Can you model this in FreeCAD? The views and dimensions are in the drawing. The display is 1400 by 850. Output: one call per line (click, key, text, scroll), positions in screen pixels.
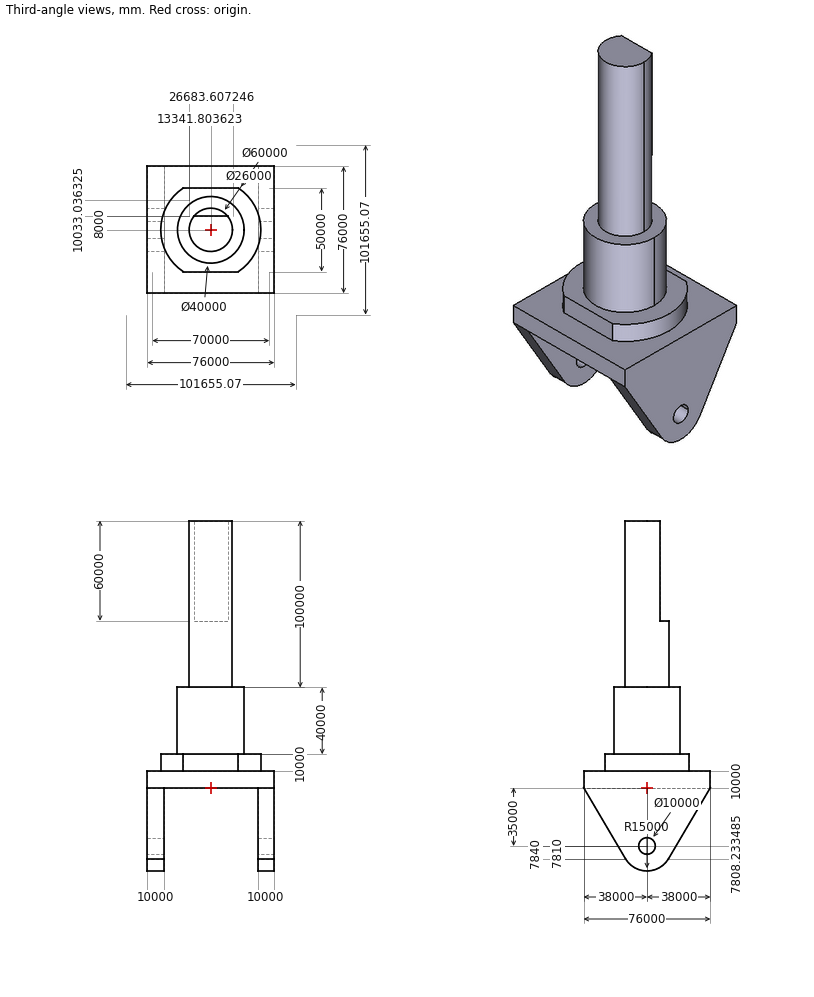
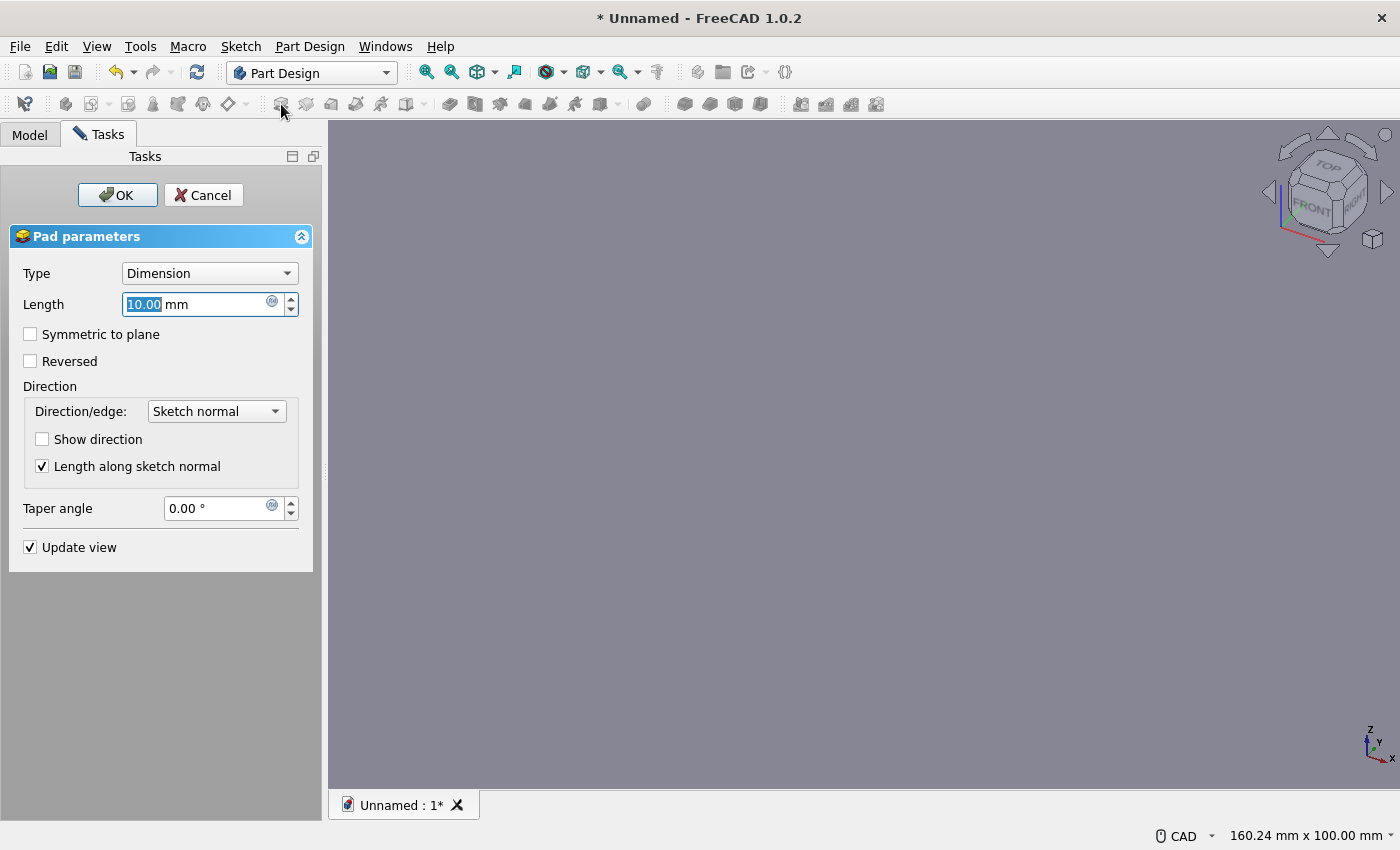
text(10000)
key(Tab)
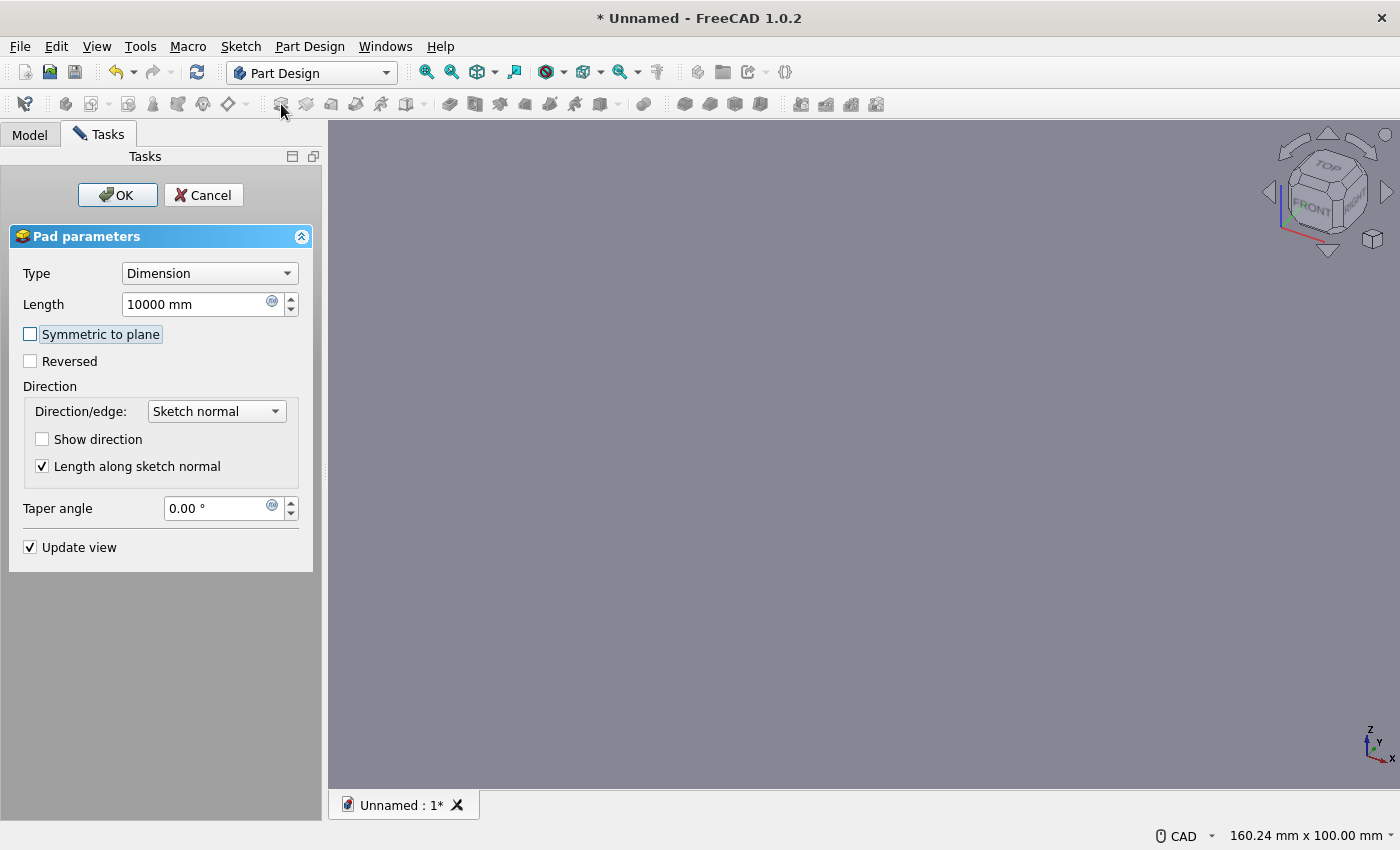
click(118, 195)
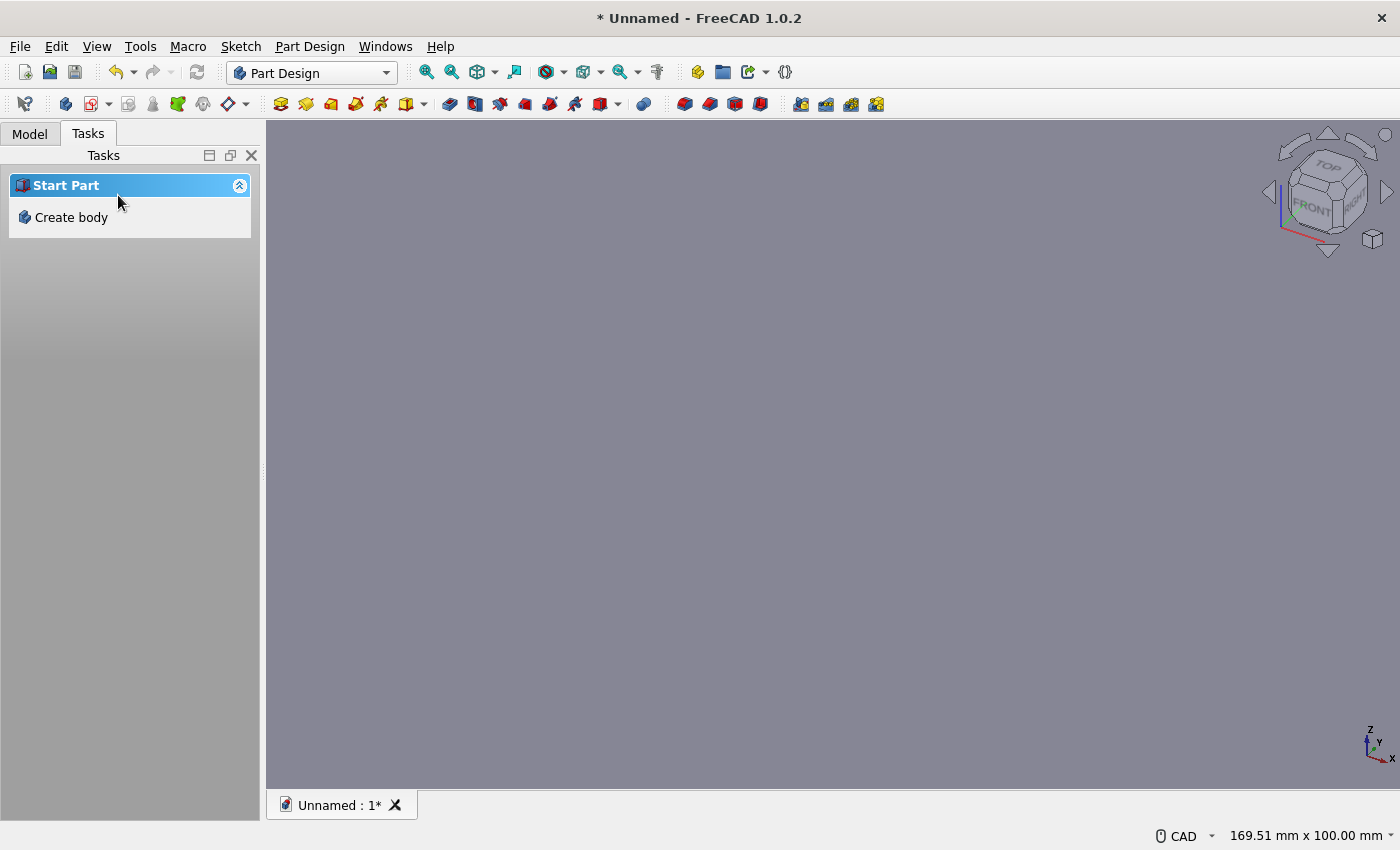
key(v)
key(f)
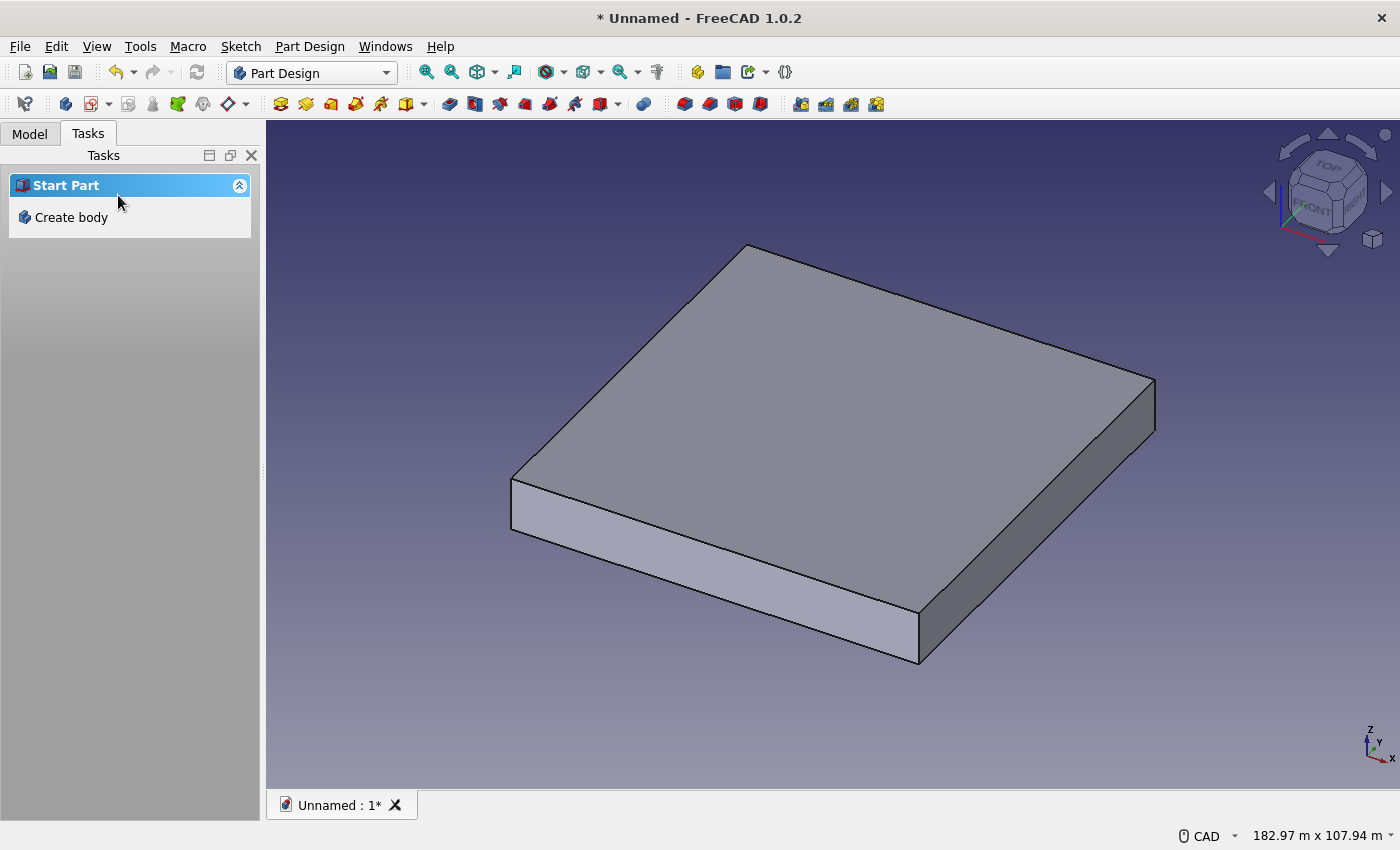
click(1138, 421)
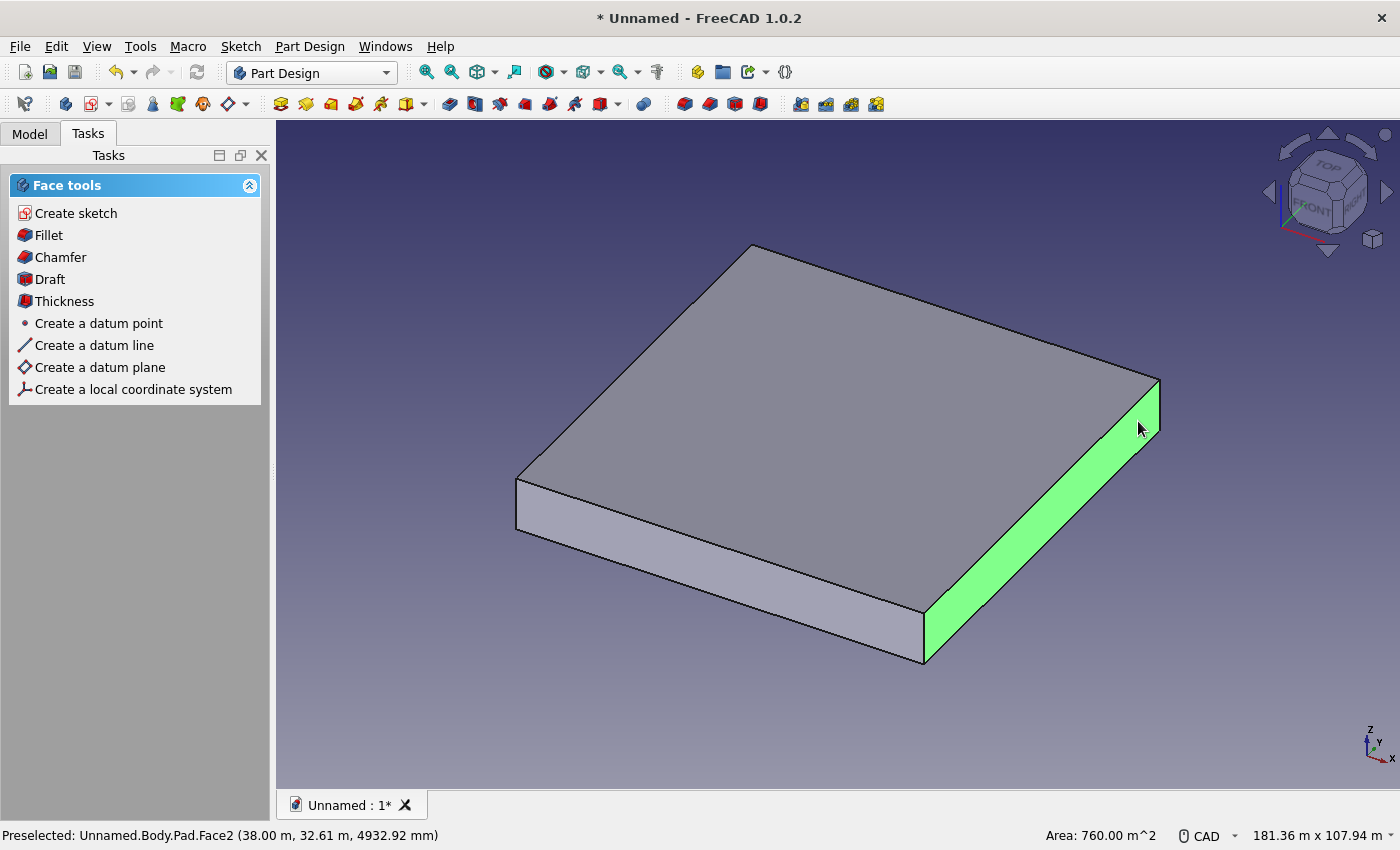
click(90, 104)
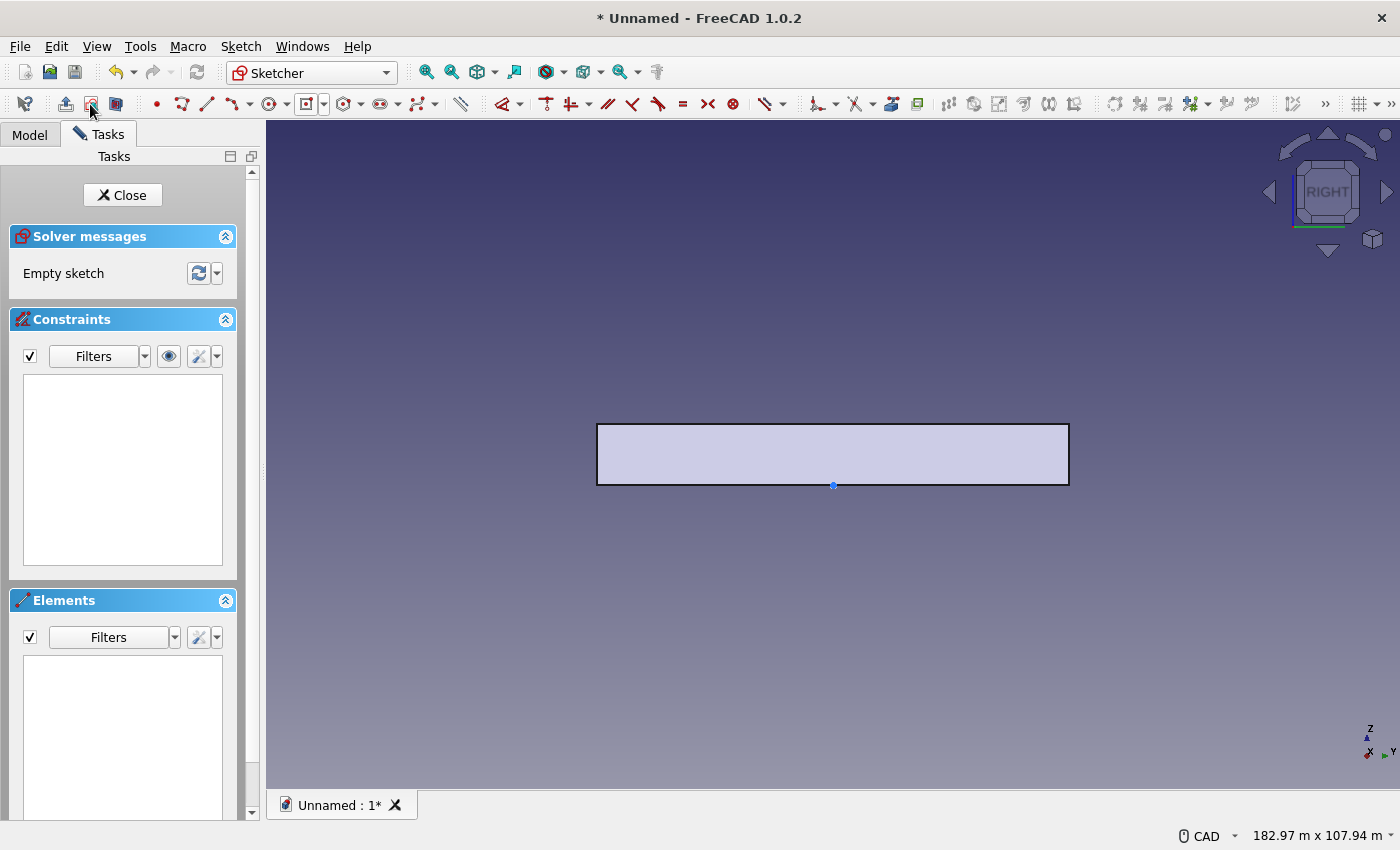
scroll(455, 148, down, 1)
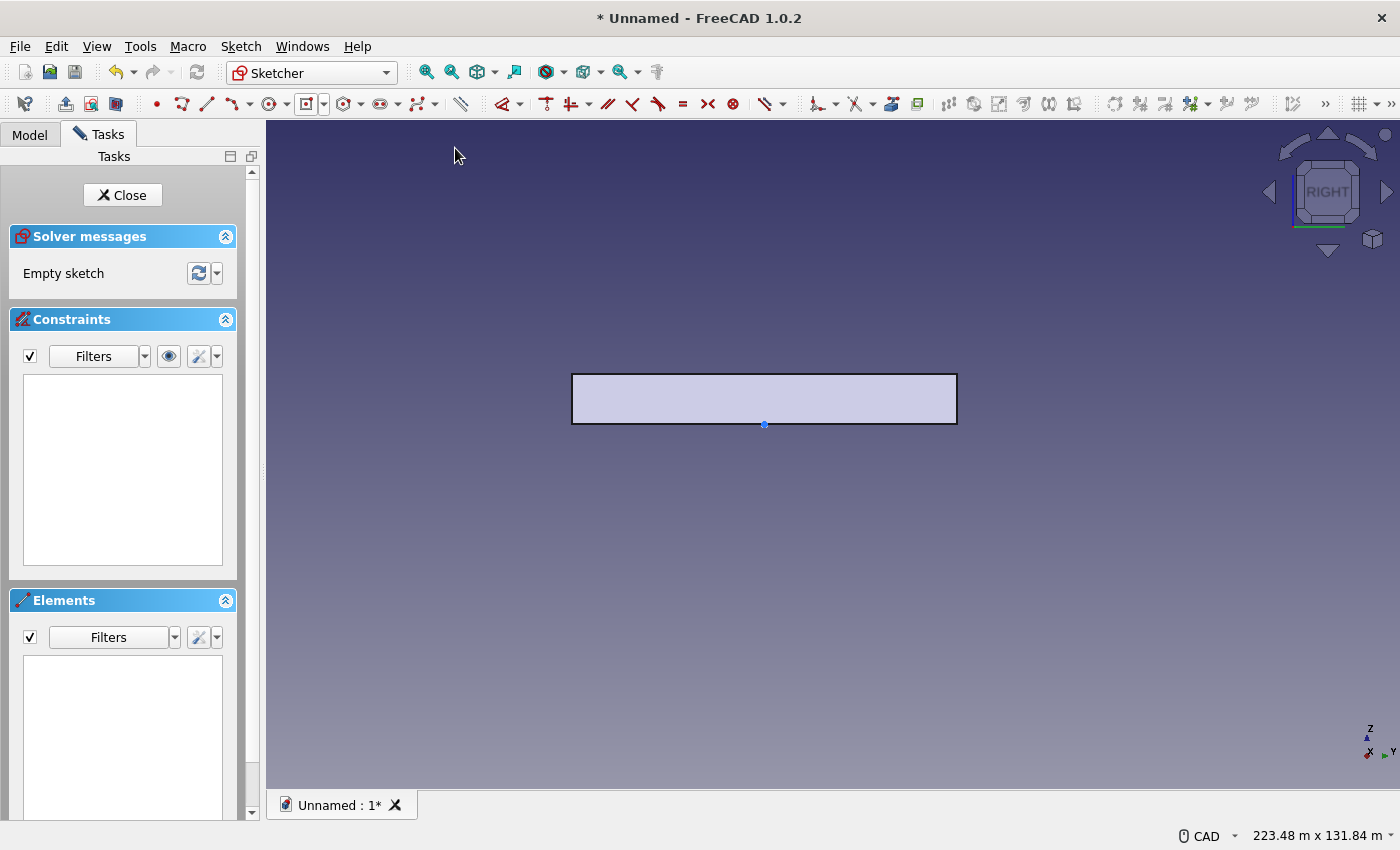
scroll(765, 669, up, 3)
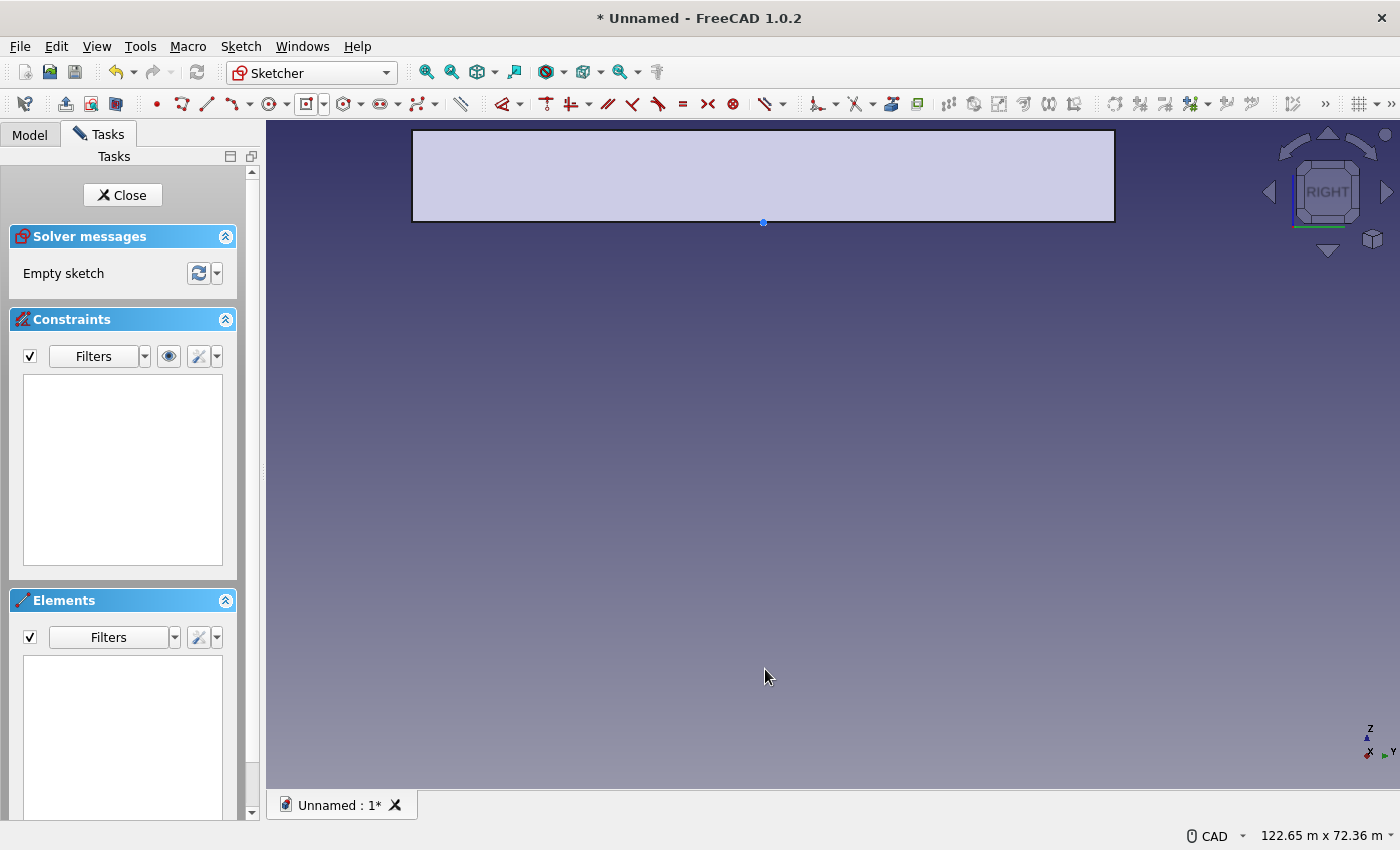
click(182, 104)